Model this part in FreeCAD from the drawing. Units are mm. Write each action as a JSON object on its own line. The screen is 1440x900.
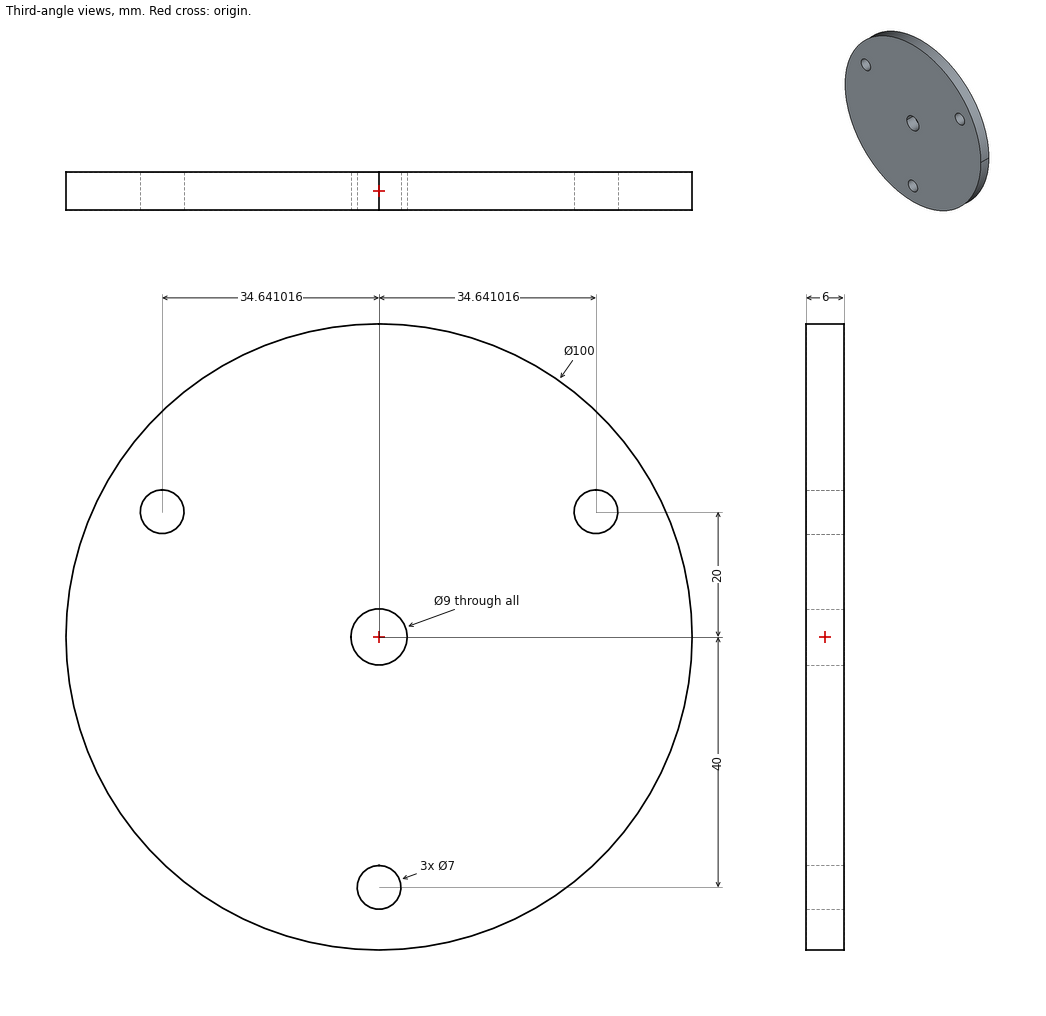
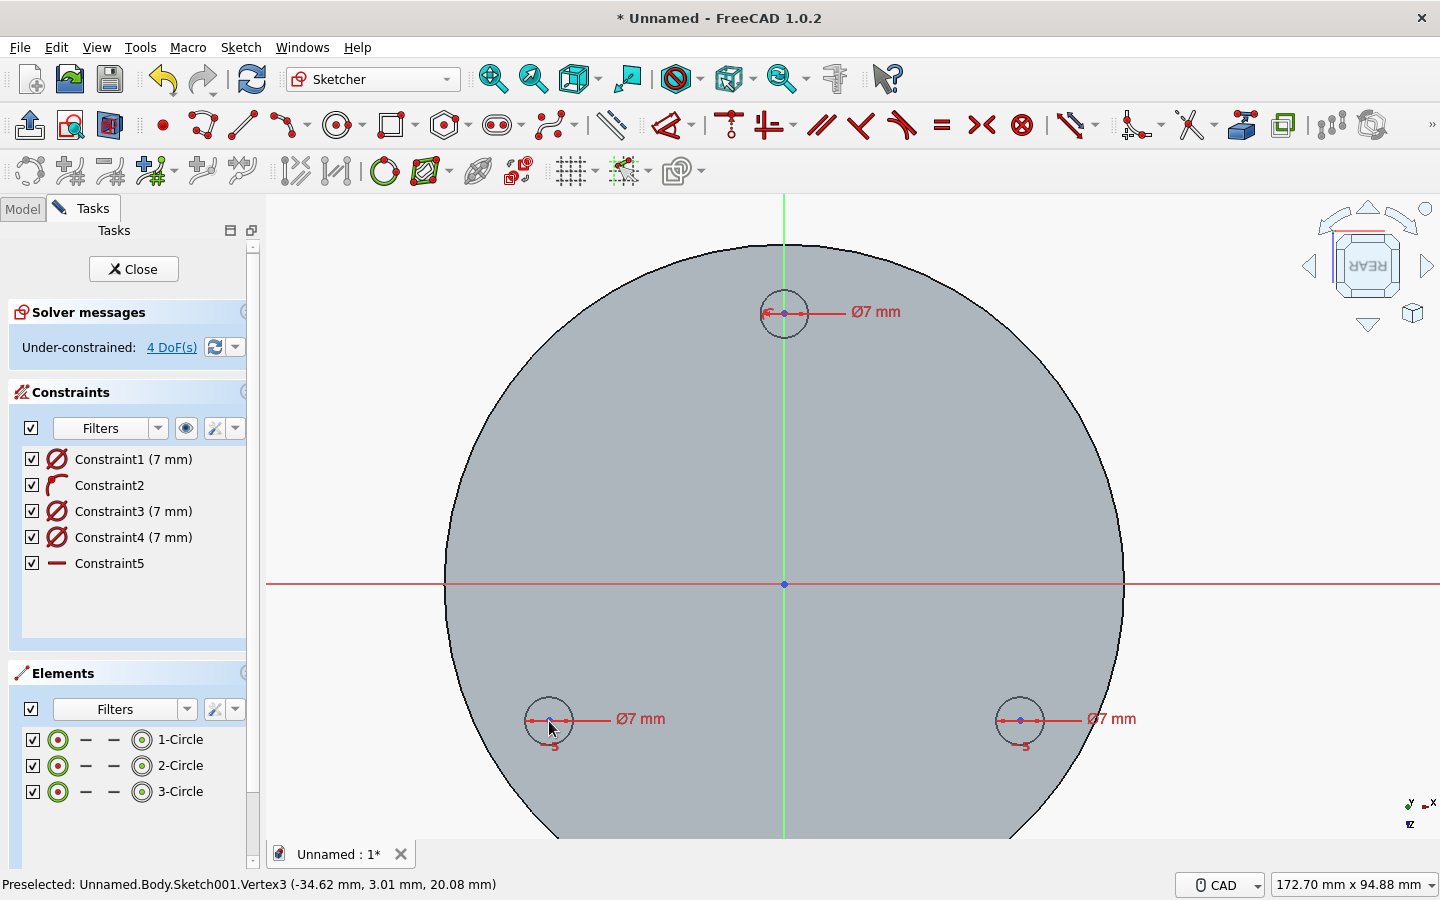
{"action": "left_click", "coordinate": [784, 314]}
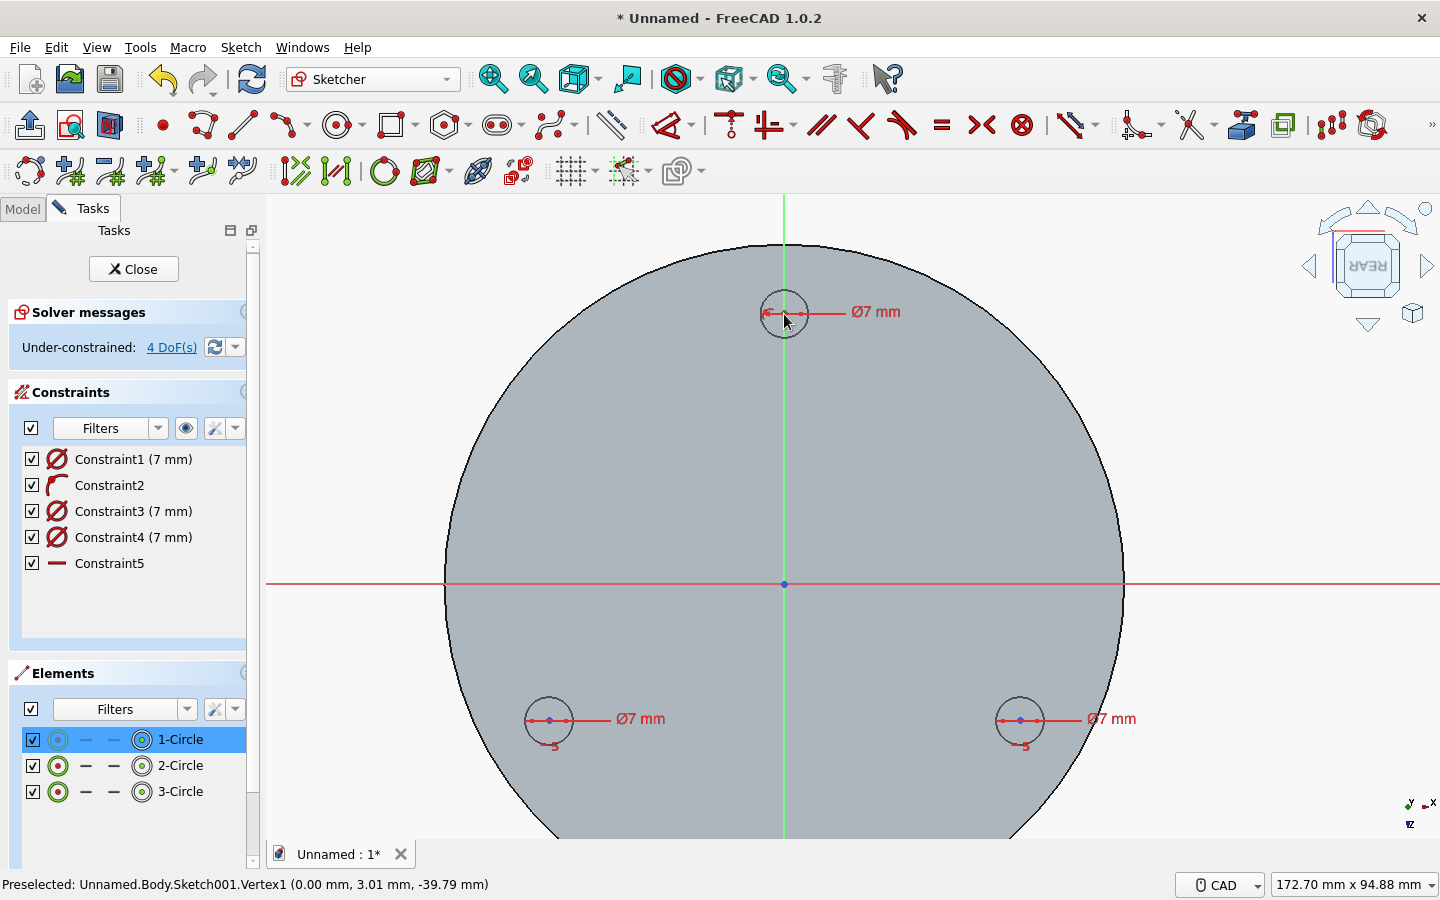
{"action": "left_click", "coordinate": [694, 126]}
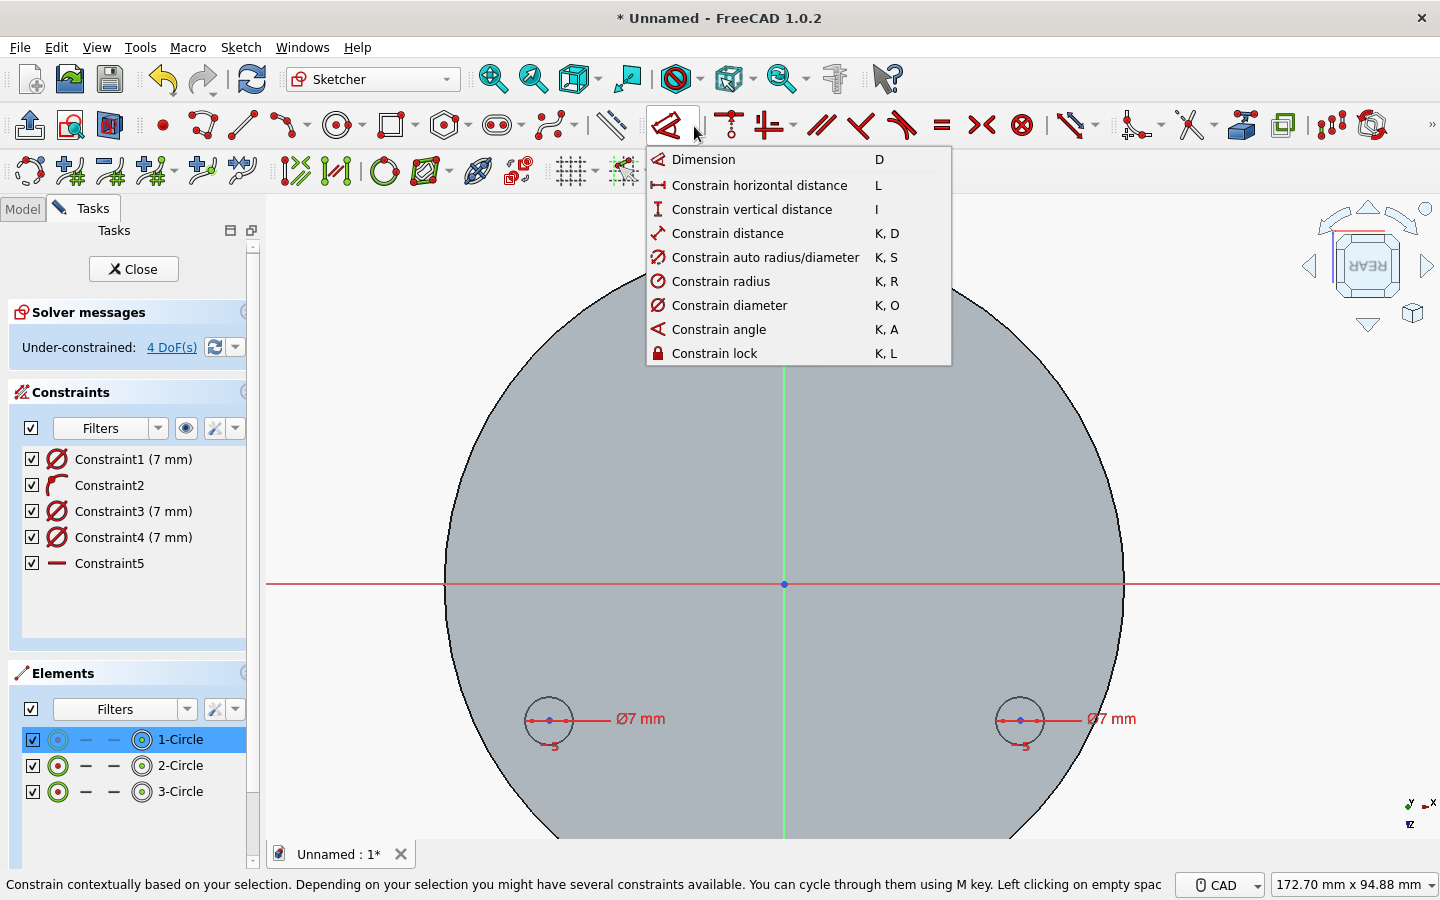
{"action": "left_click", "coordinate": [799, 209]}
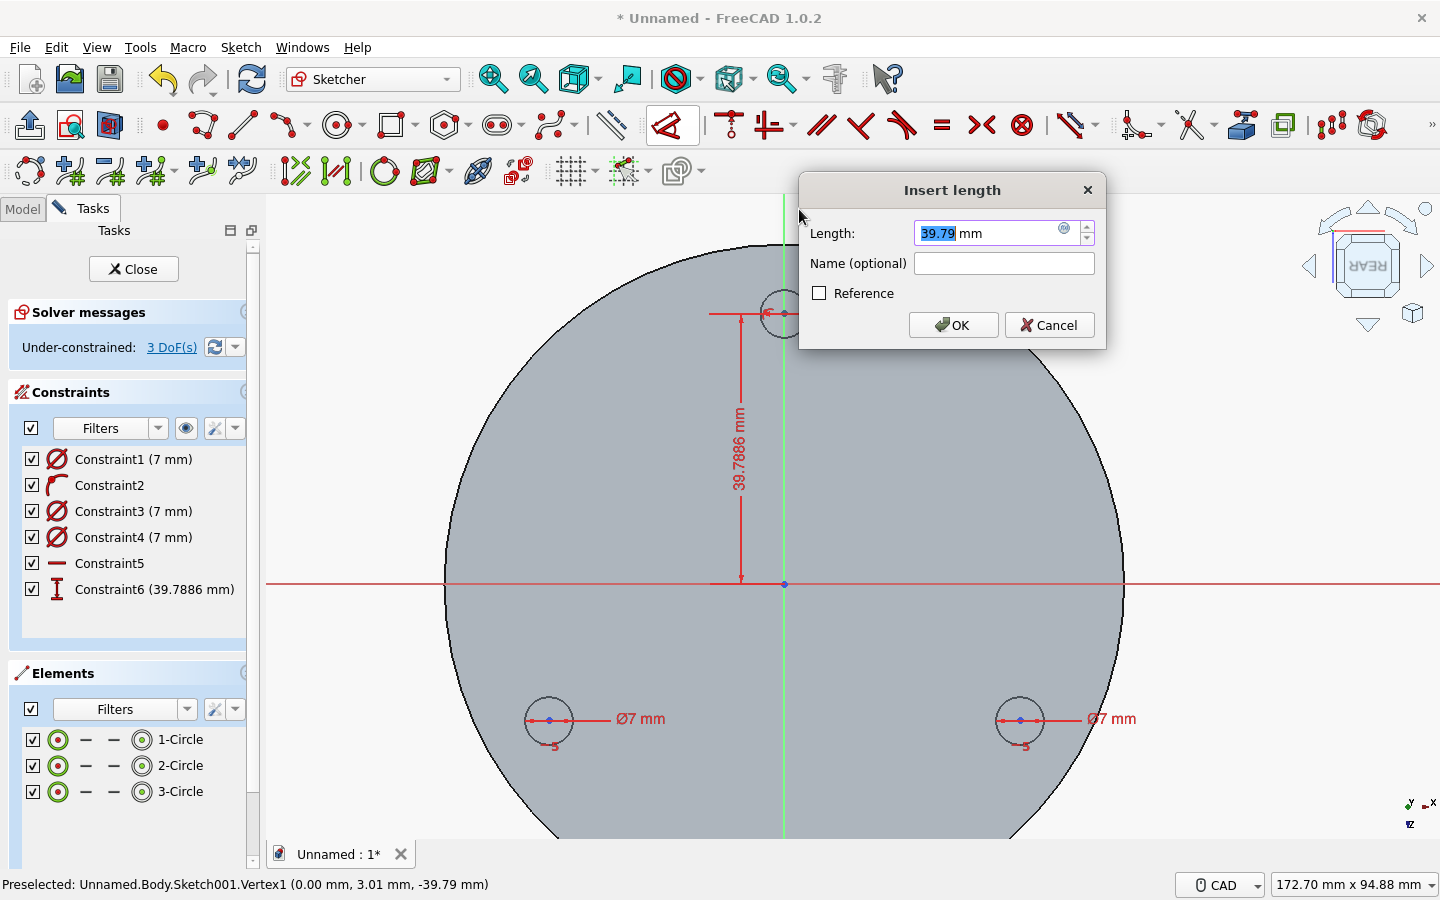
{"action": "type", "text": "40"}
{"action": "key", "text": "Return"}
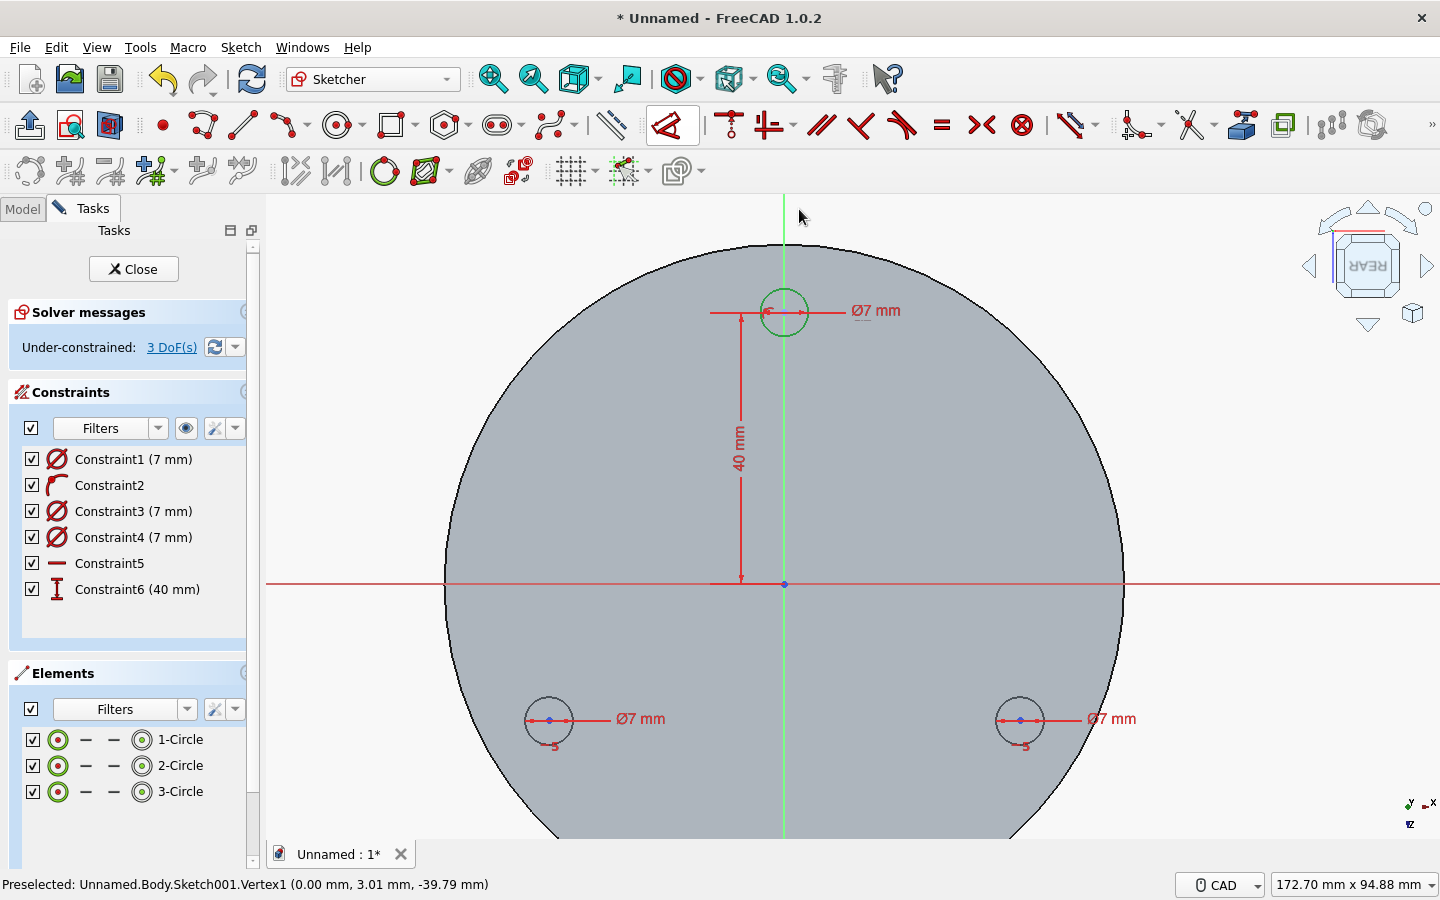
{"action": "left_click", "coordinate": [1020, 721]}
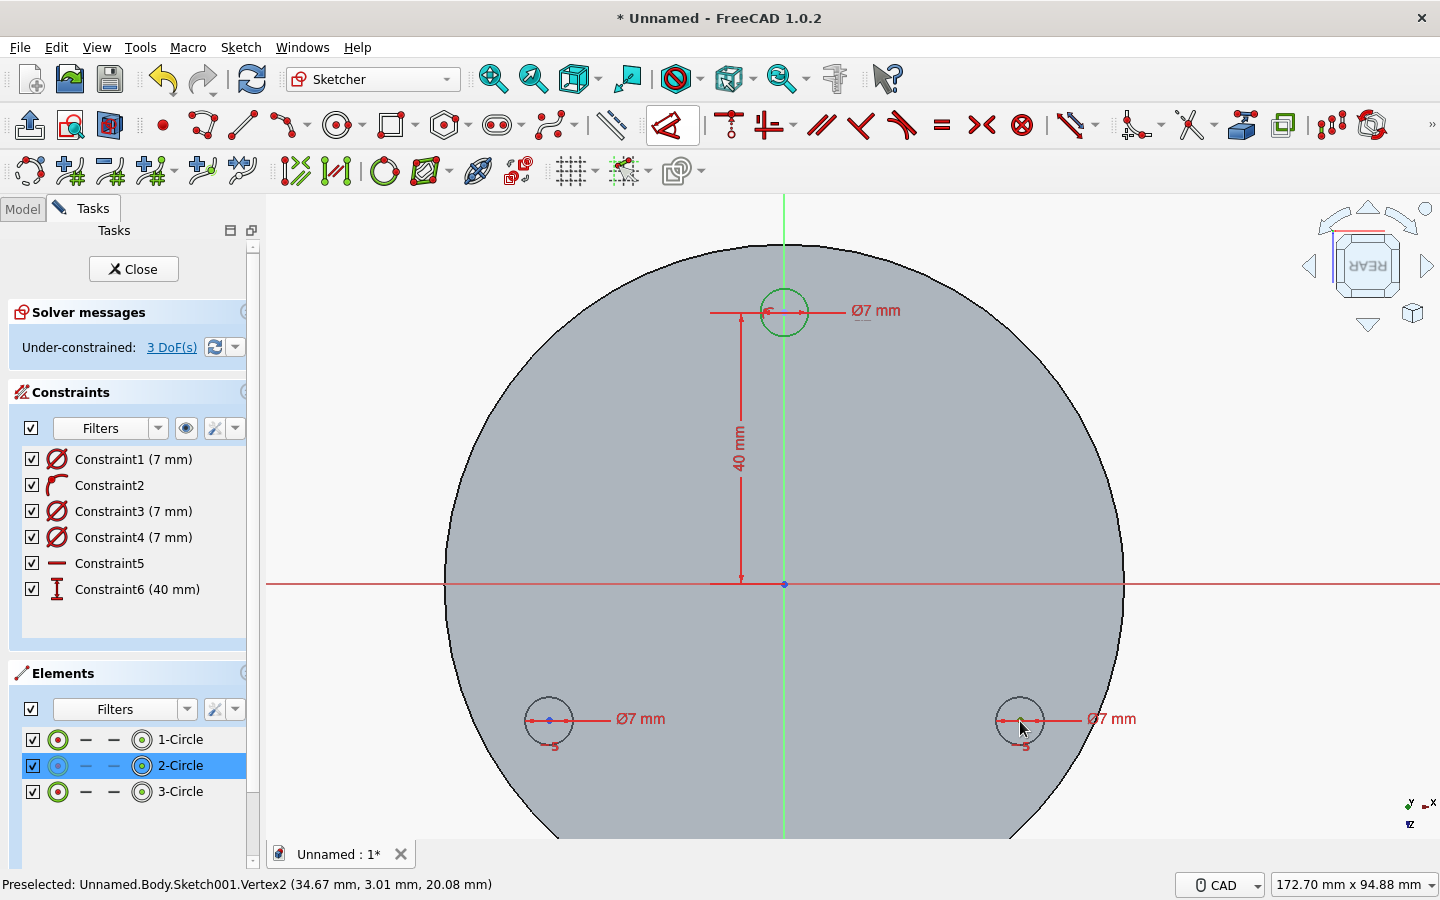
{"action": "key", "text": "i"}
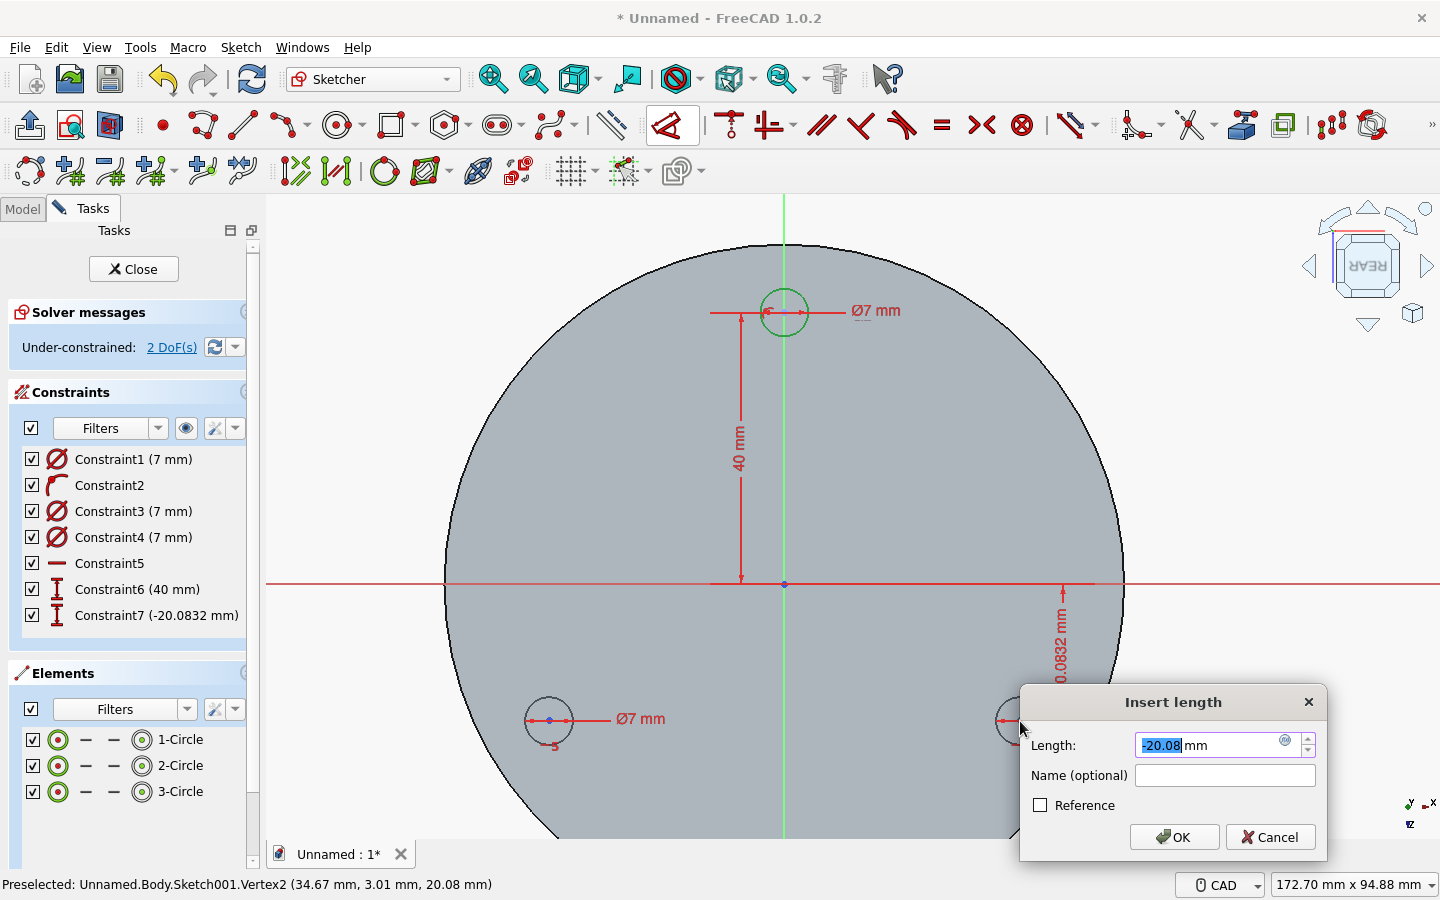
{"action": "type", "text": "-20"}
{"action": "key", "text": "Return"}